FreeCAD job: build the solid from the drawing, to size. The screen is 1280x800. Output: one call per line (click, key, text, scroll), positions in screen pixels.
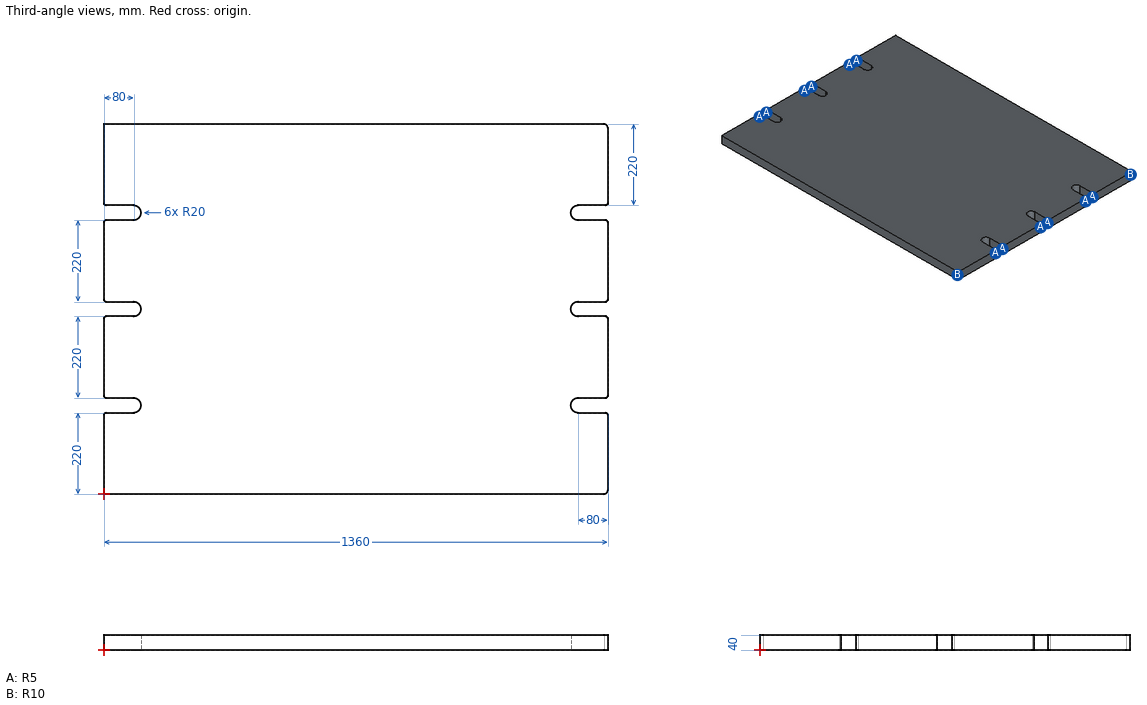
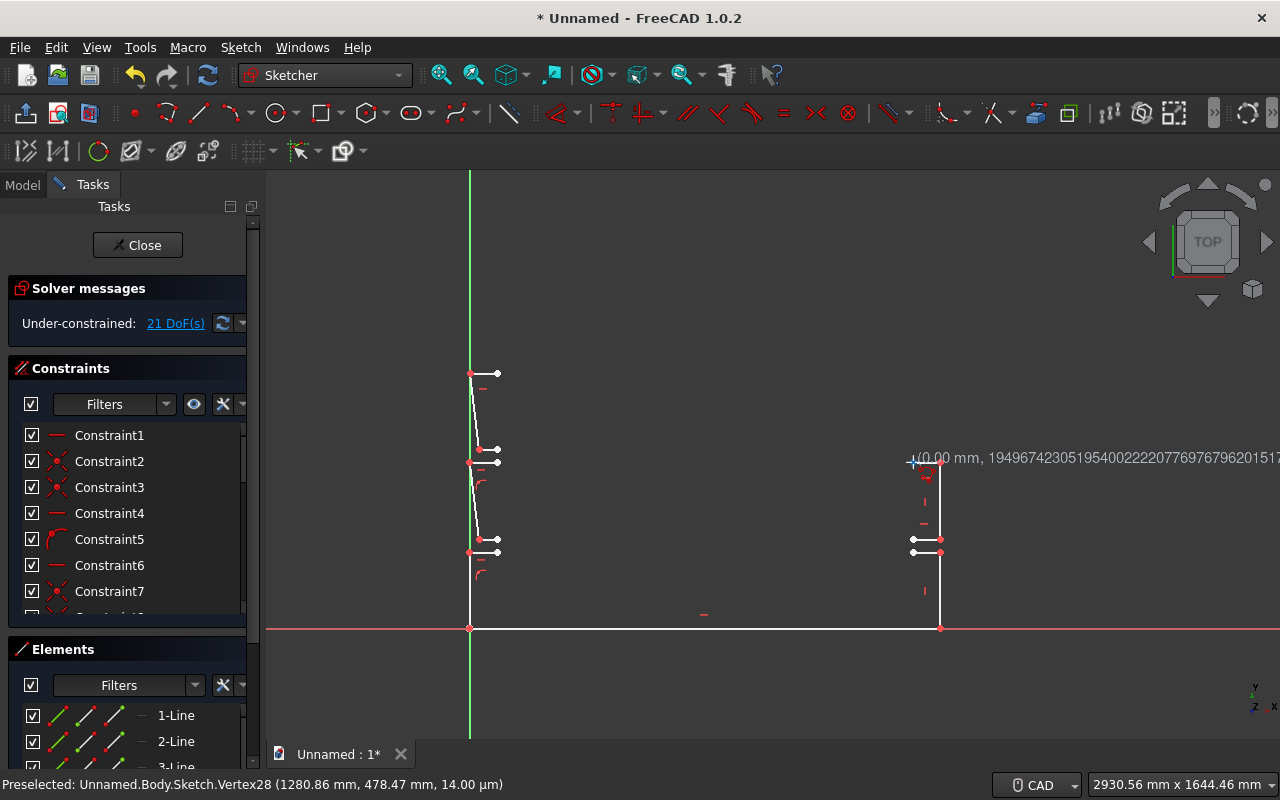
click(913, 449)
click(940, 449)
click(940, 373)
click(913, 373)
right_click(913, 373)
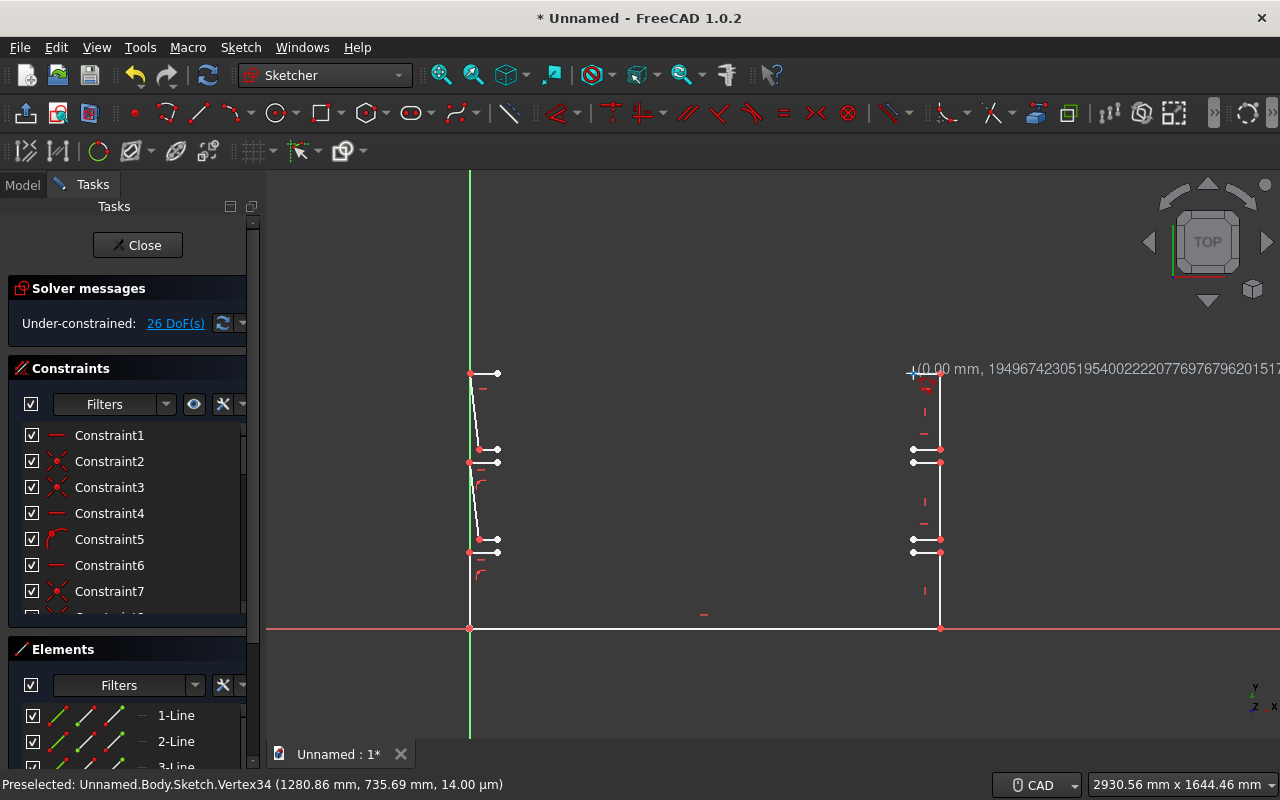
click(913, 359)
click(940, 359)
click(940, 283)
click(470, 283)
click(479, 359)
click(497, 359)
right_click(497, 359)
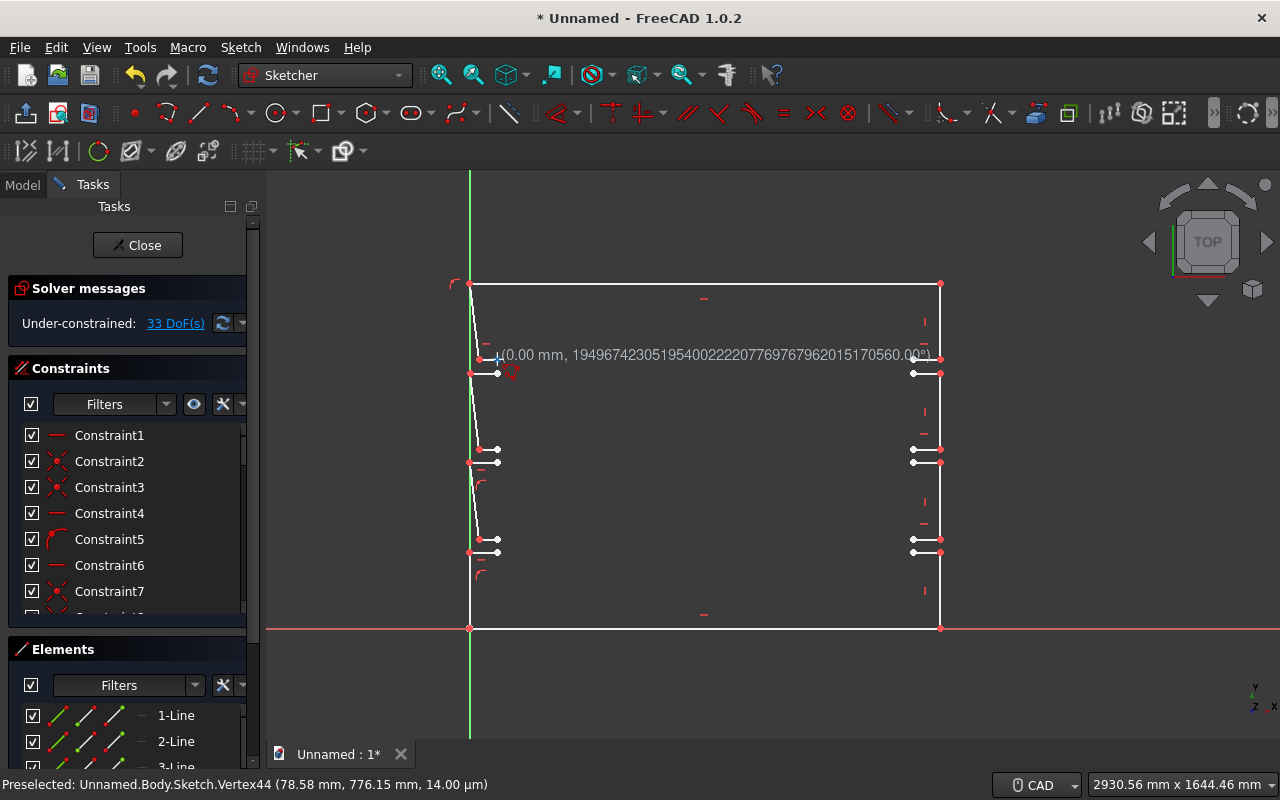
click(232, 114)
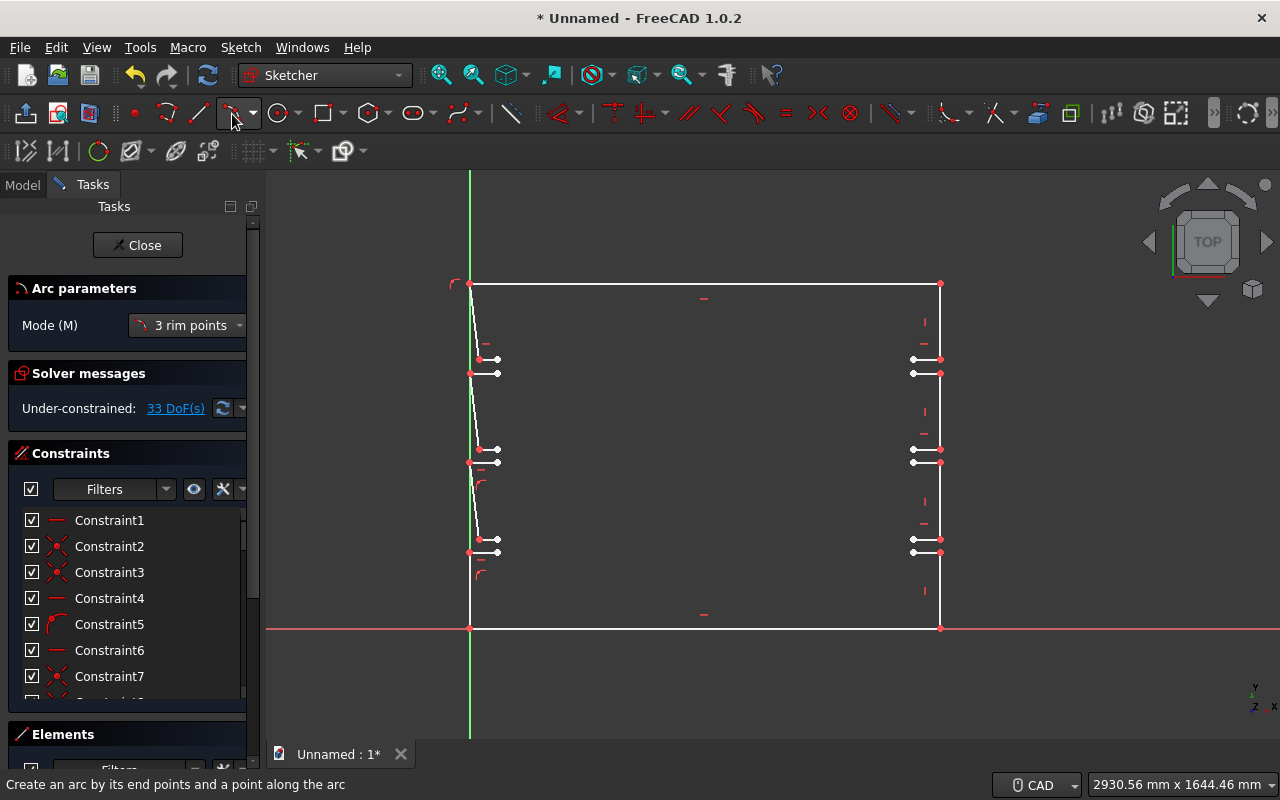
click(497, 450)
click(497, 463)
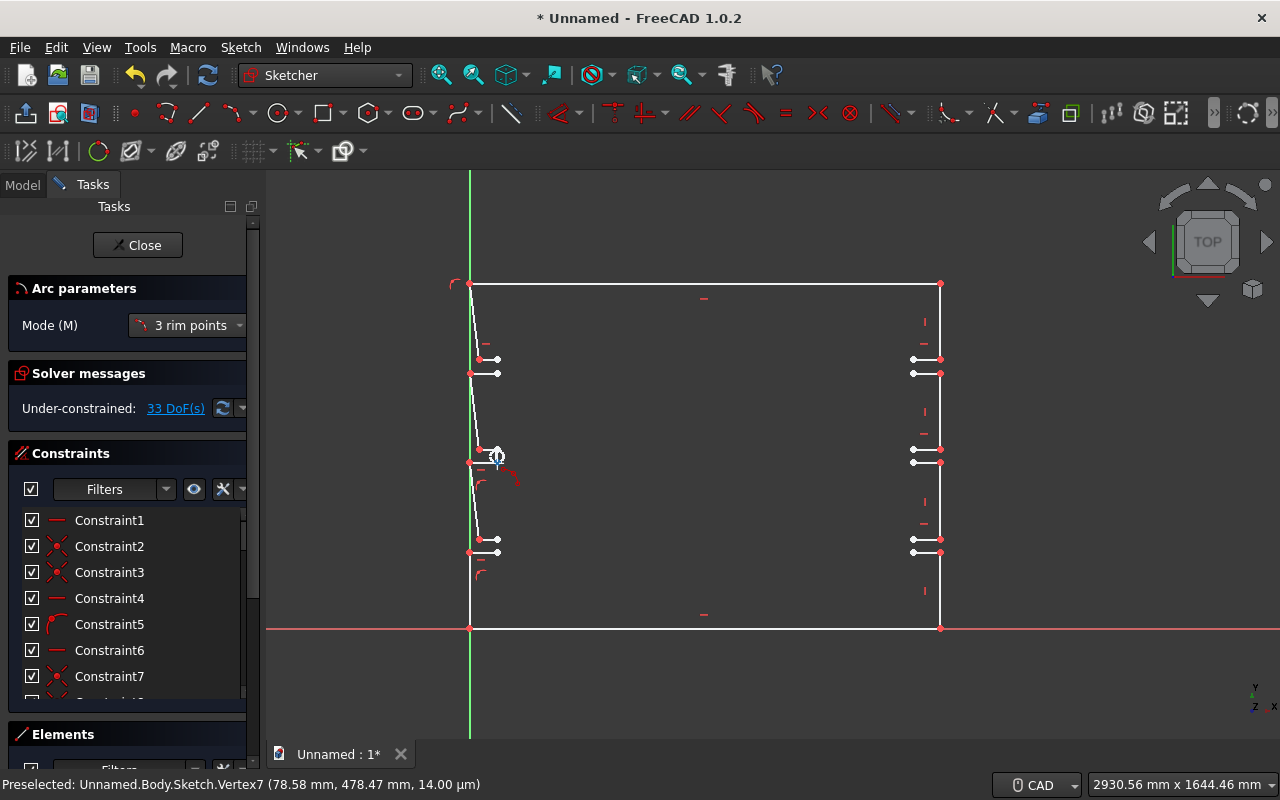
scroll(504, 456, up, 5)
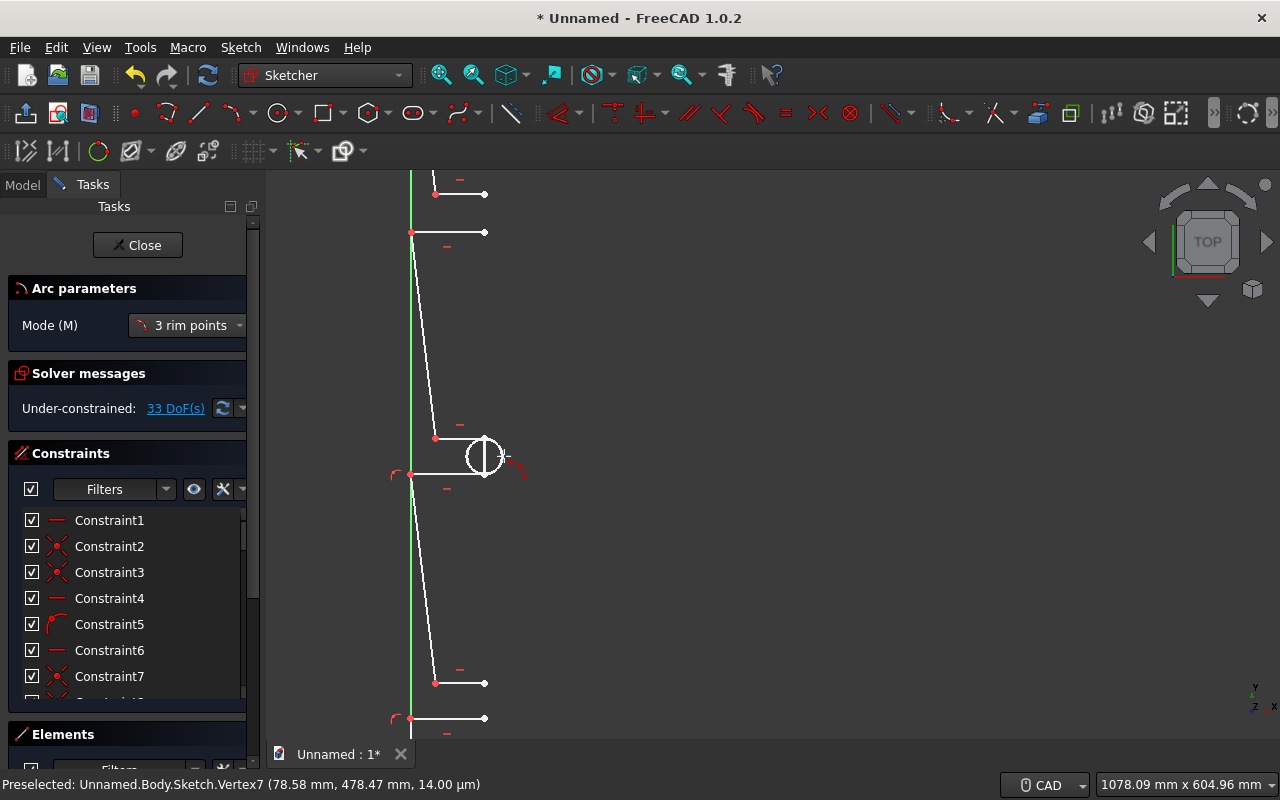
click(505, 454)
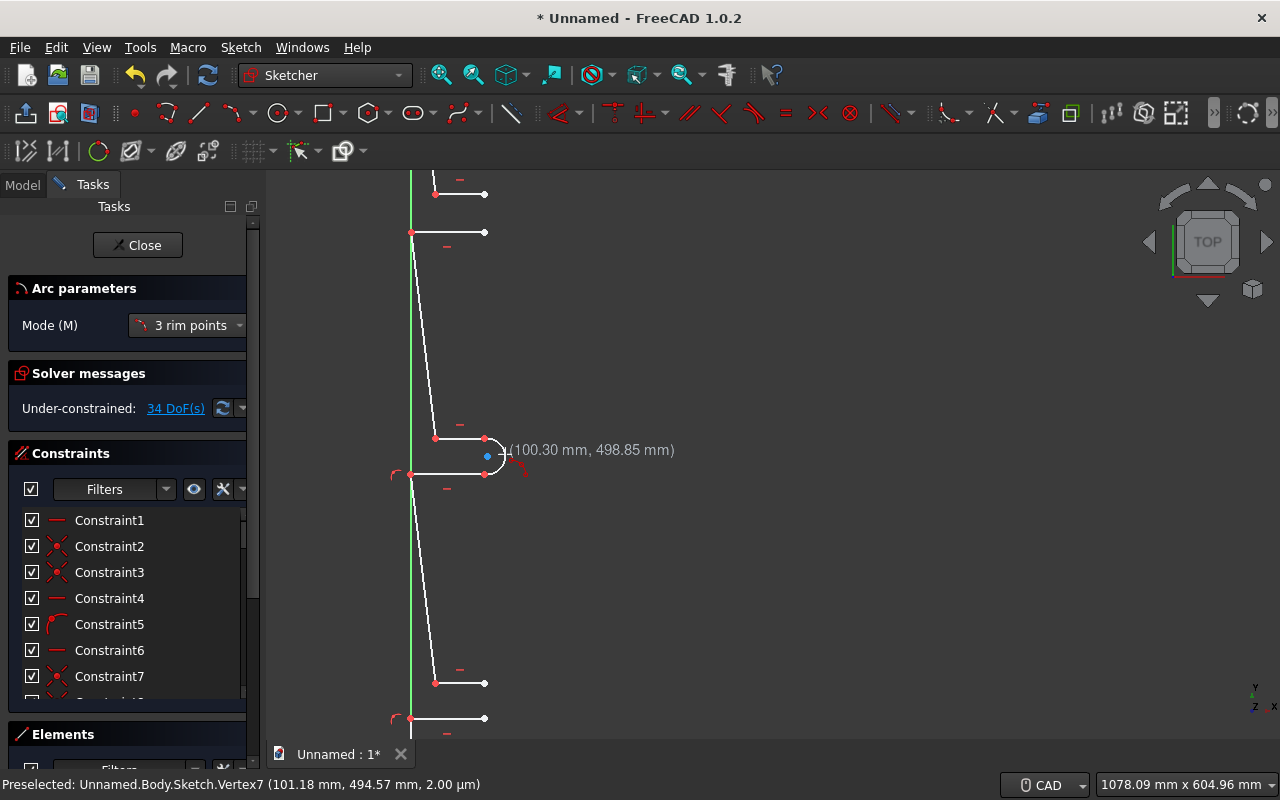
click(485, 683)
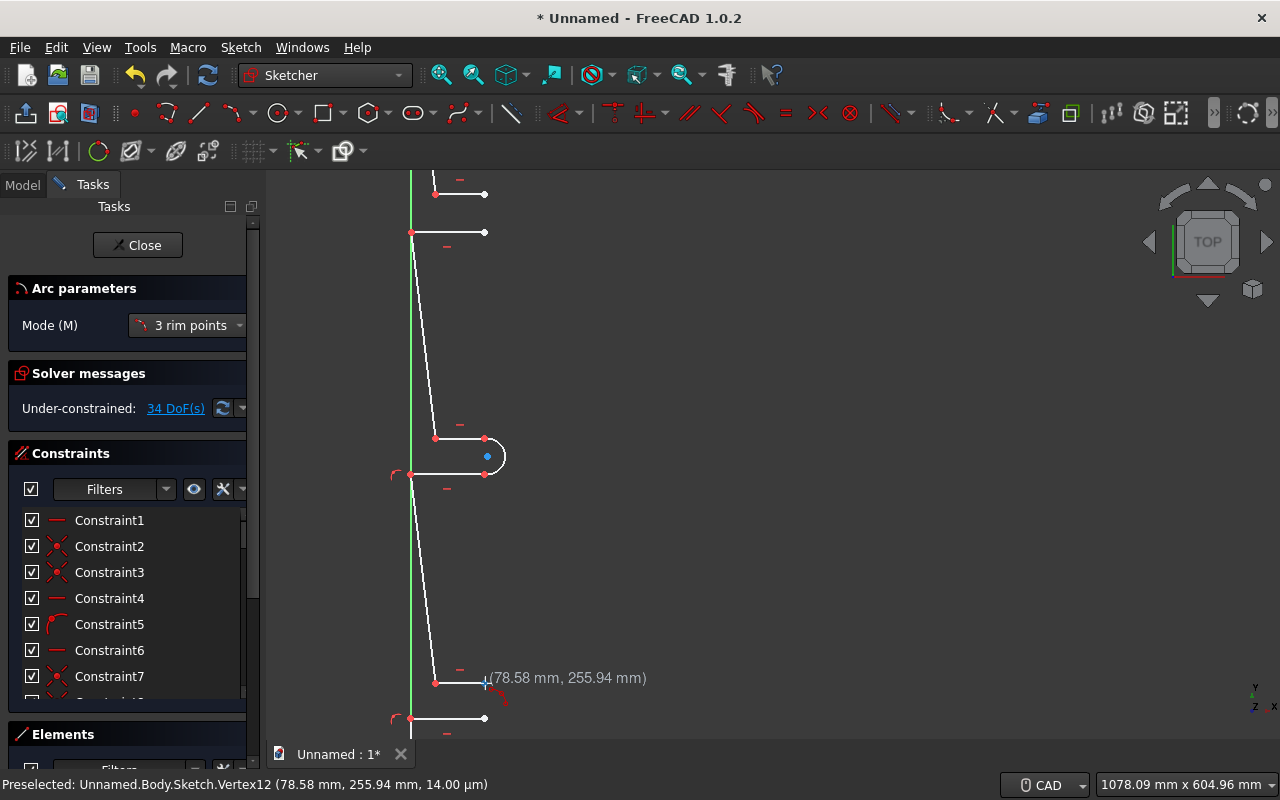
scroll(503, 455, down, 5)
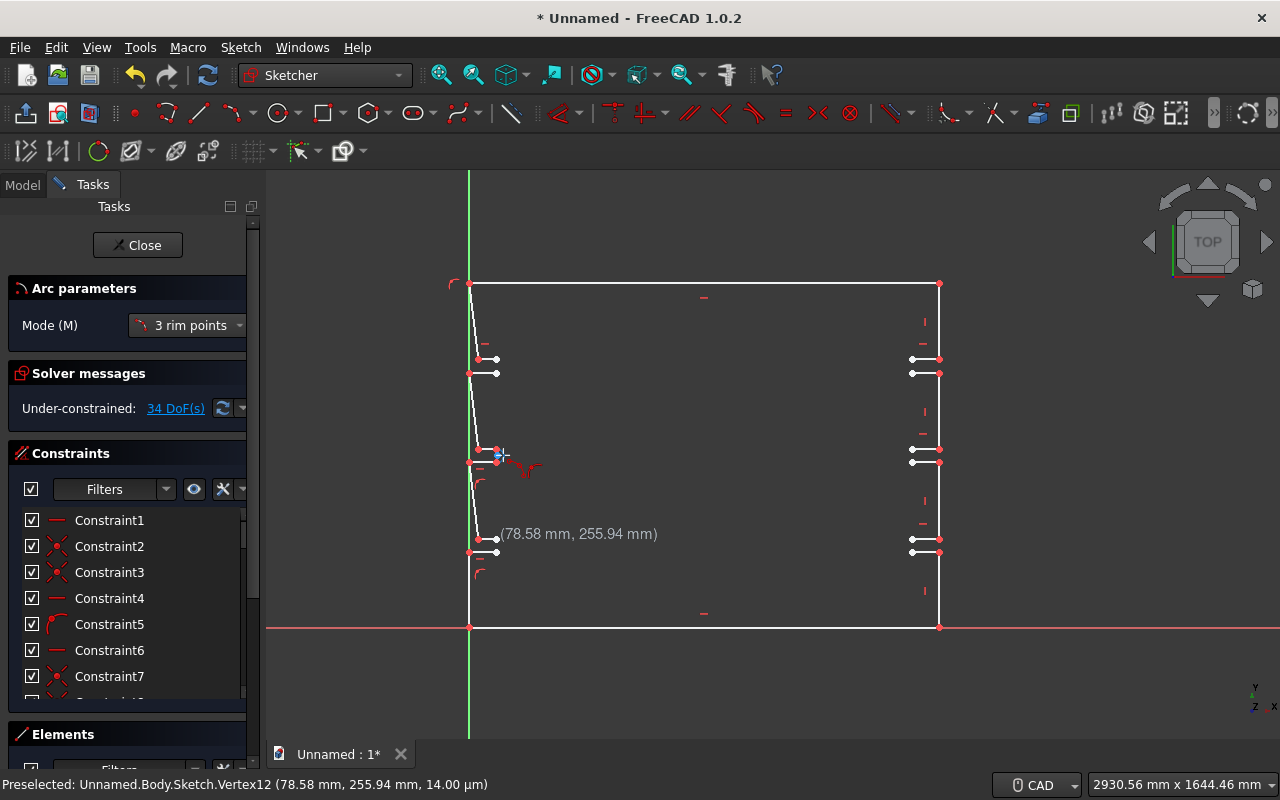
click(496, 552)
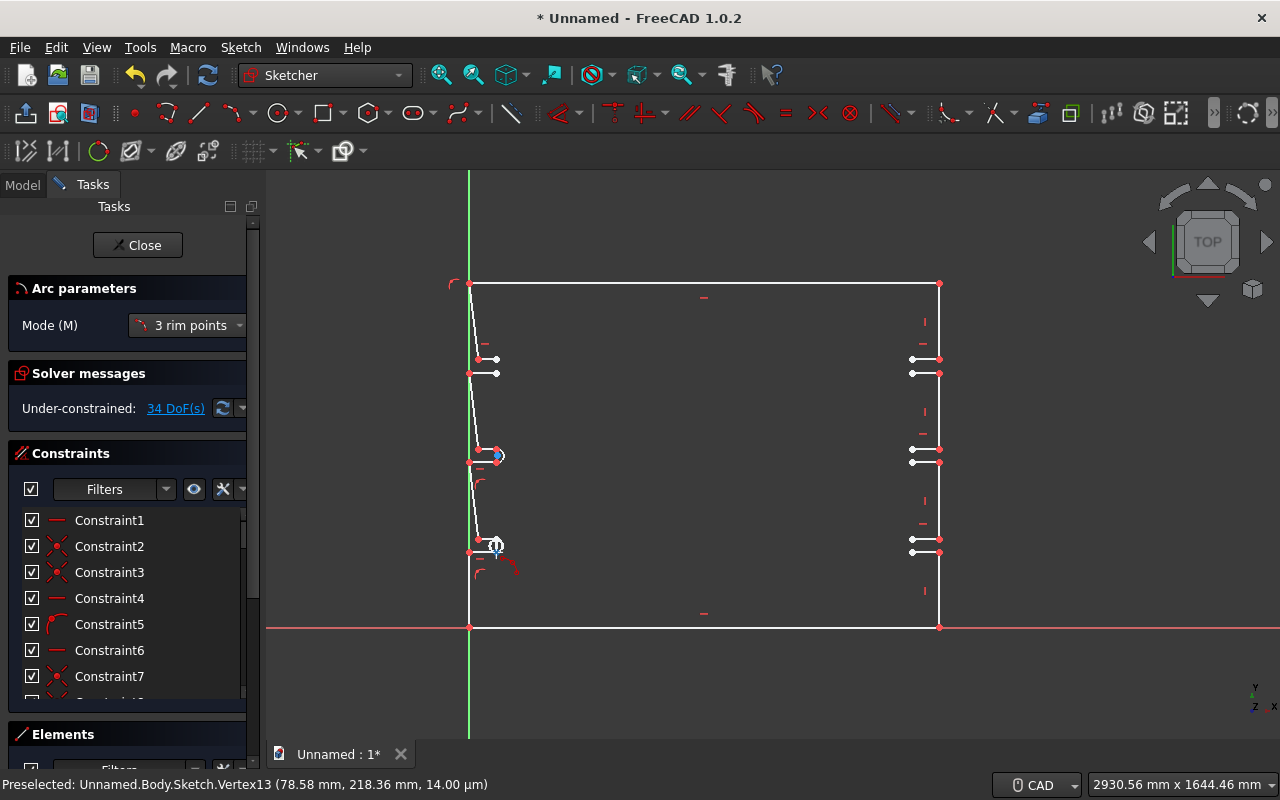
scroll(504, 545, up, 5)